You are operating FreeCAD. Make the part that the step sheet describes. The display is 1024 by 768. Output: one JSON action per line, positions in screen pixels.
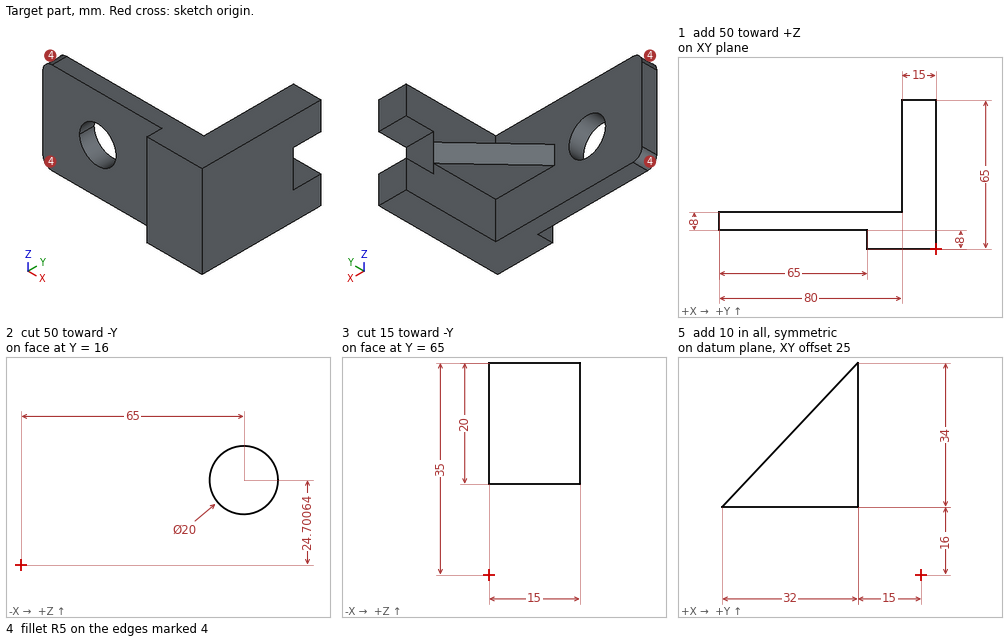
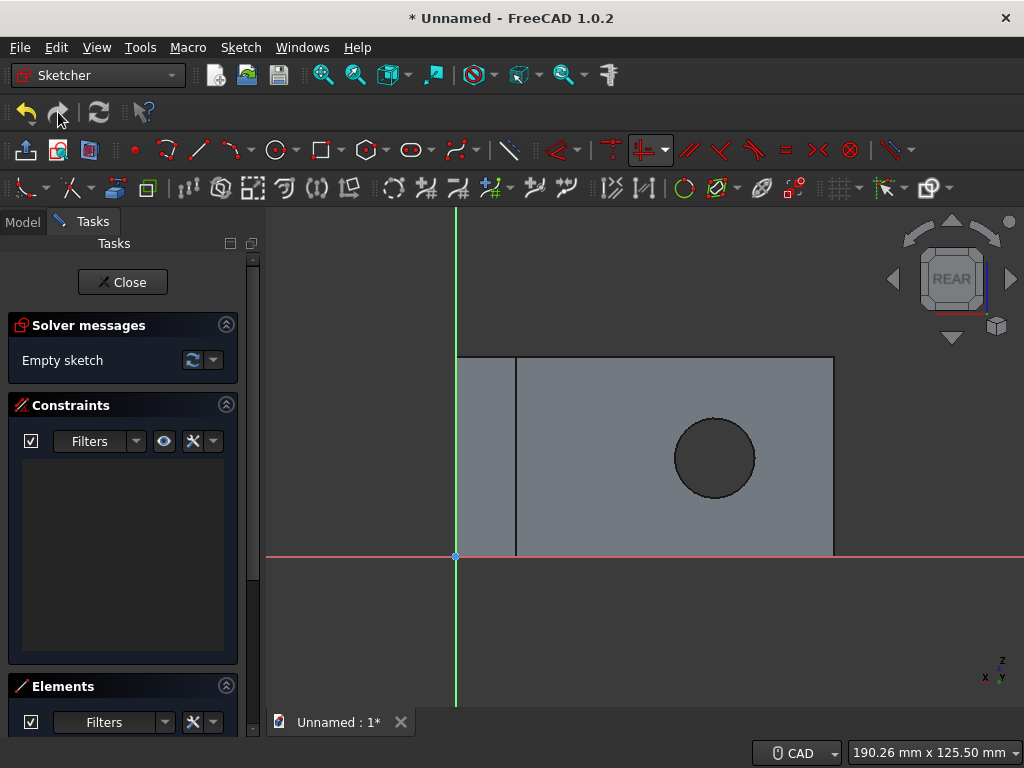
{"action": "scroll", "coordinate": [411, 511], "scroll_direction": "up", "scroll_amount": 4}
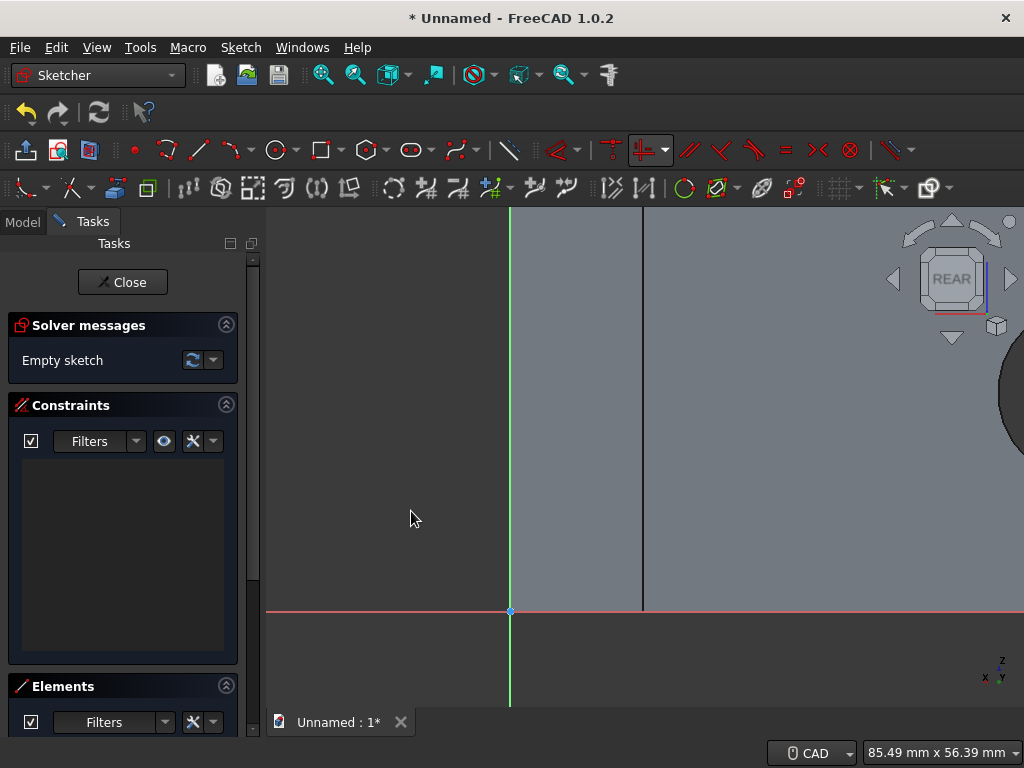
{"action": "left_click", "coordinate": [322, 150]}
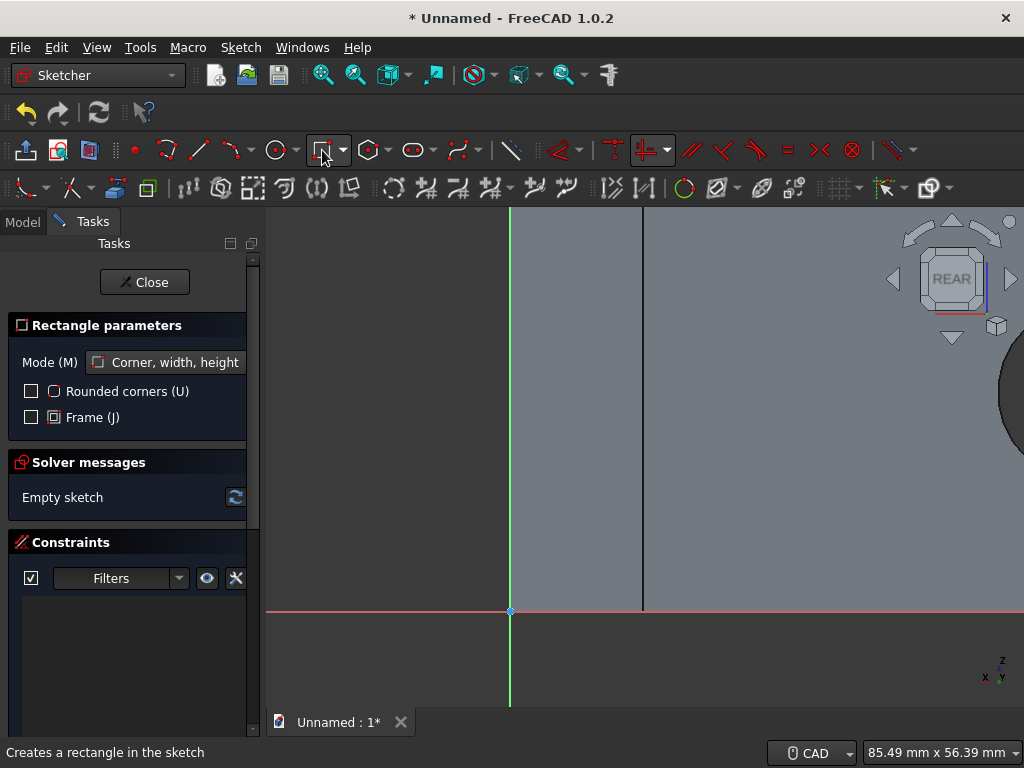
{"action": "left_click", "coordinate": [510, 301]}
{"action": "left_click", "coordinate": [643, 479]}
{"action": "key", "text": "Escape"}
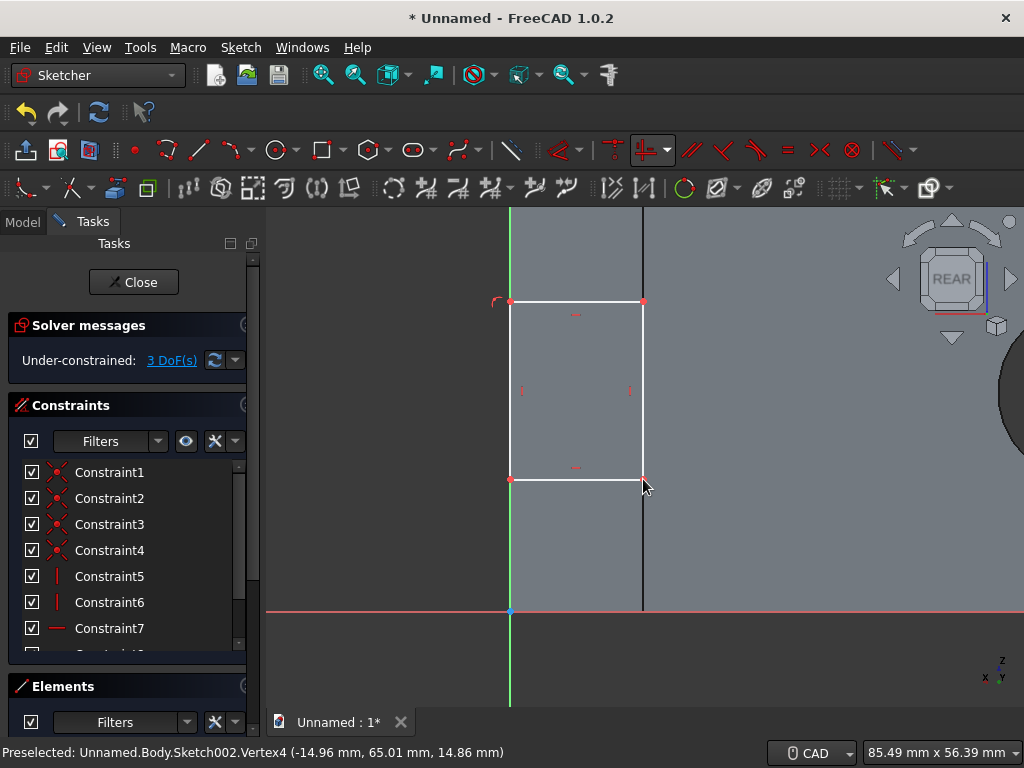
{"action": "left_click", "coordinate": [558, 150]}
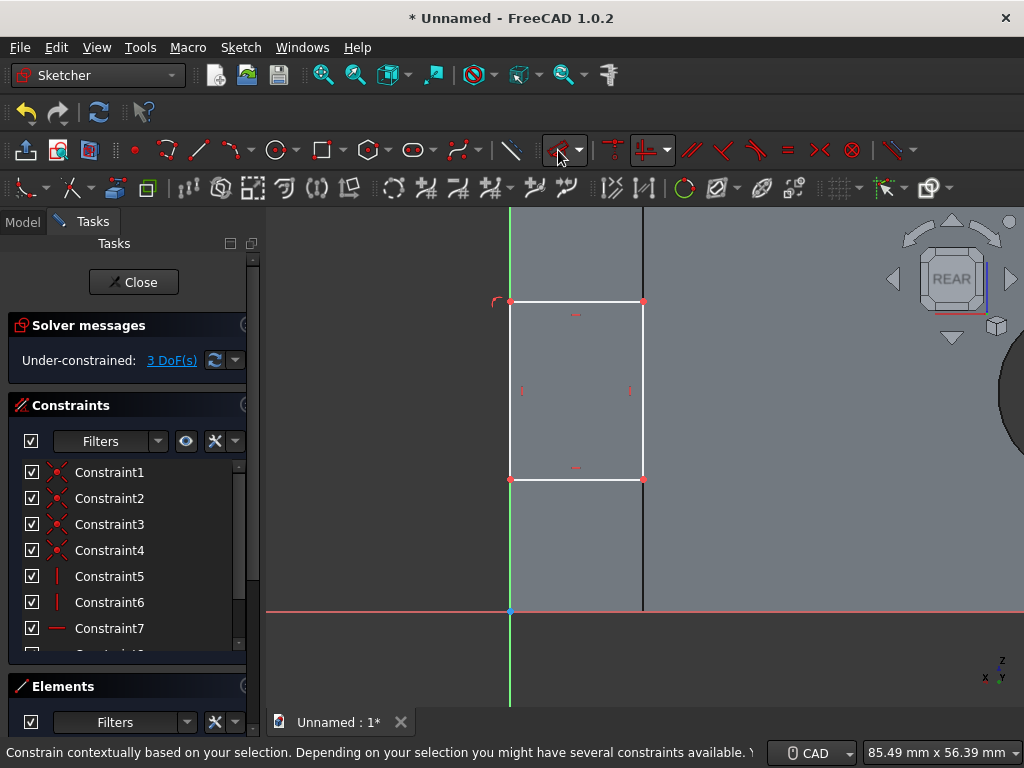
{"action": "left_click", "coordinate": [510, 355]}
{"action": "left_click", "coordinate": [476, 391]}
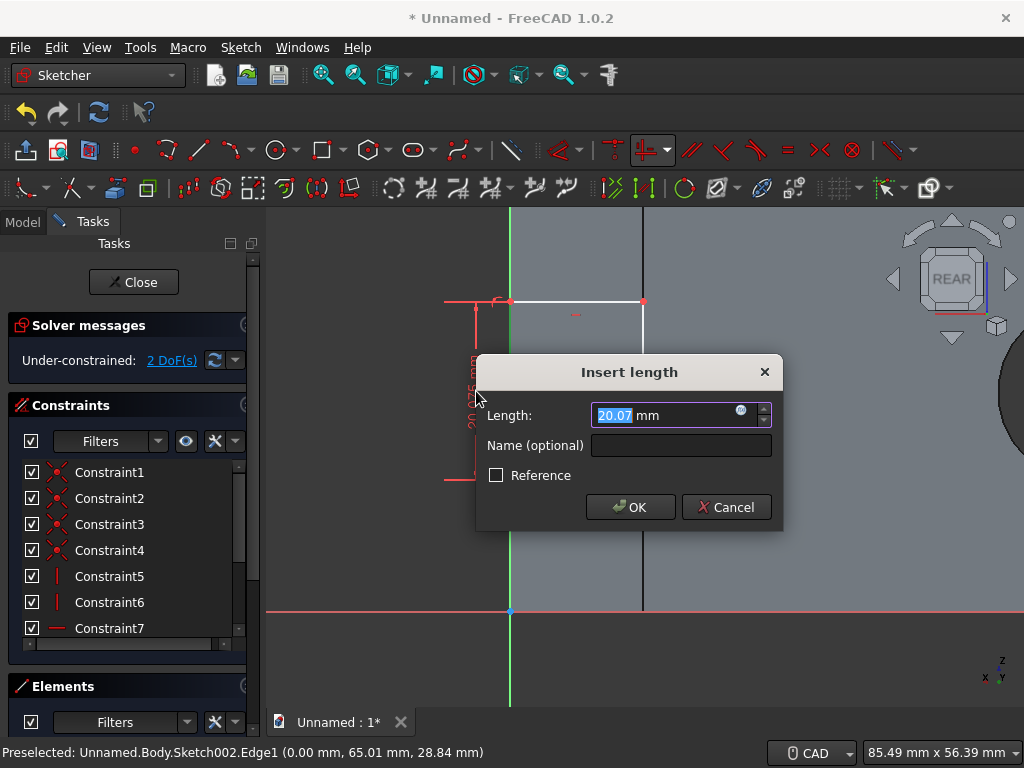
{"action": "type", "text": "20"}
{"action": "key", "text": "Return"}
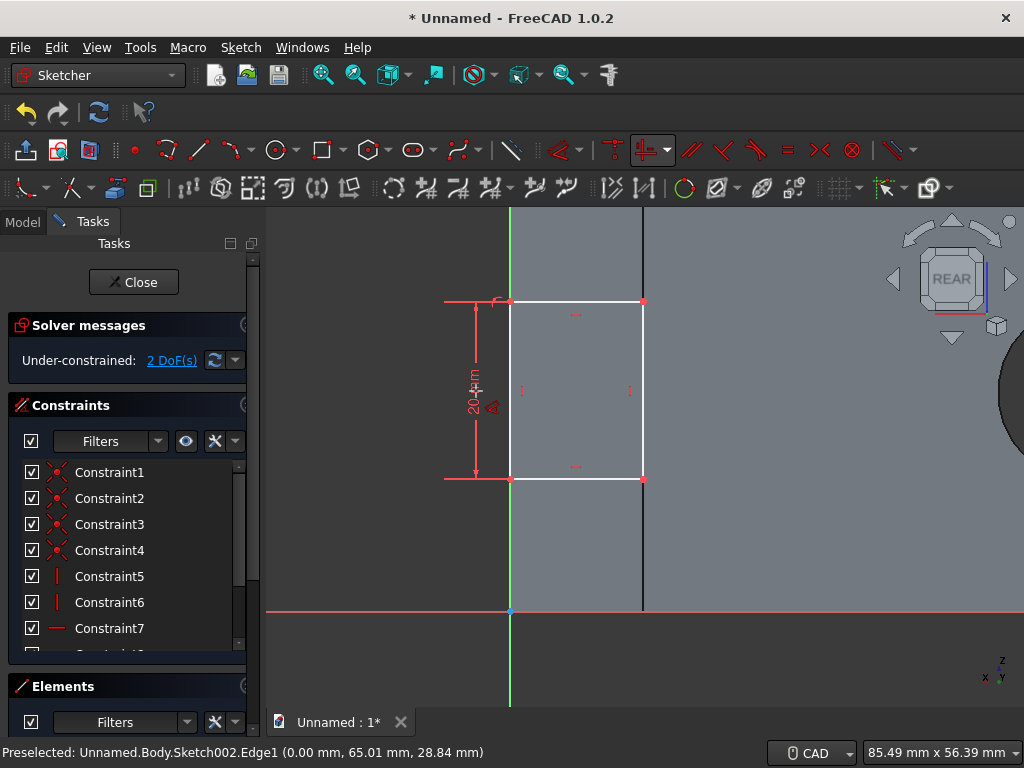
{"action": "left_click", "coordinate": [550, 479]}
{"action": "left_click", "coordinate": [577, 513]}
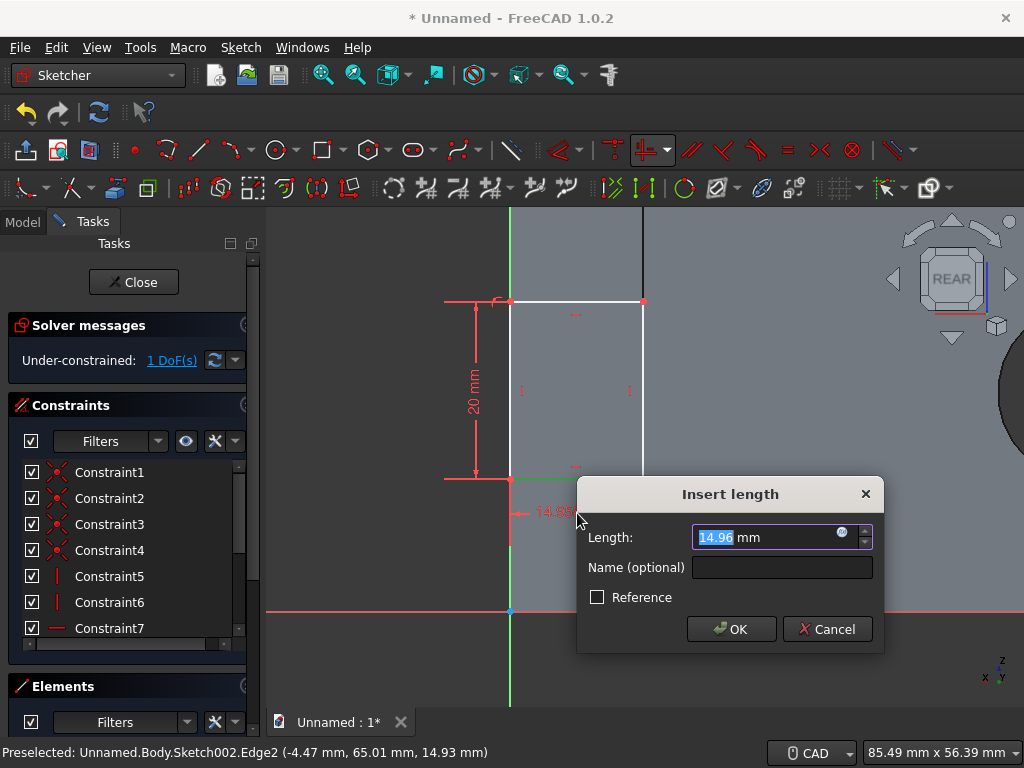
{"action": "type", "text": "15"}
{"action": "key", "text": "Return"}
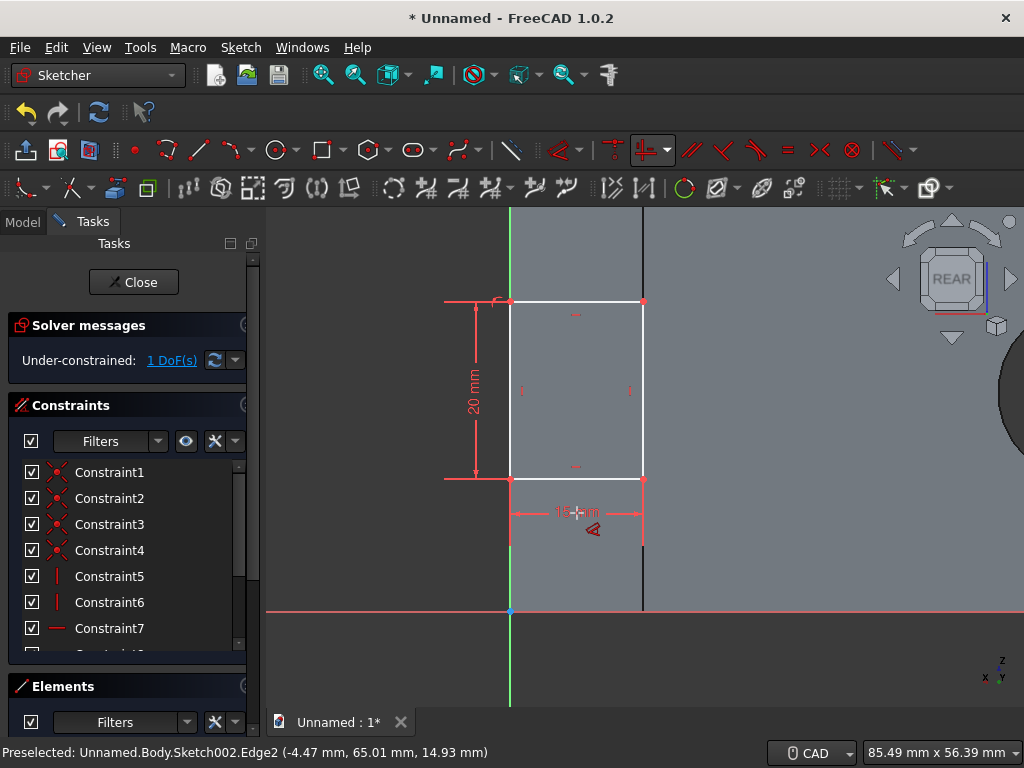
{"action": "left_click", "coordinate": [510, 302]}
{"action": "left_click", "coordinate": [476, 457]}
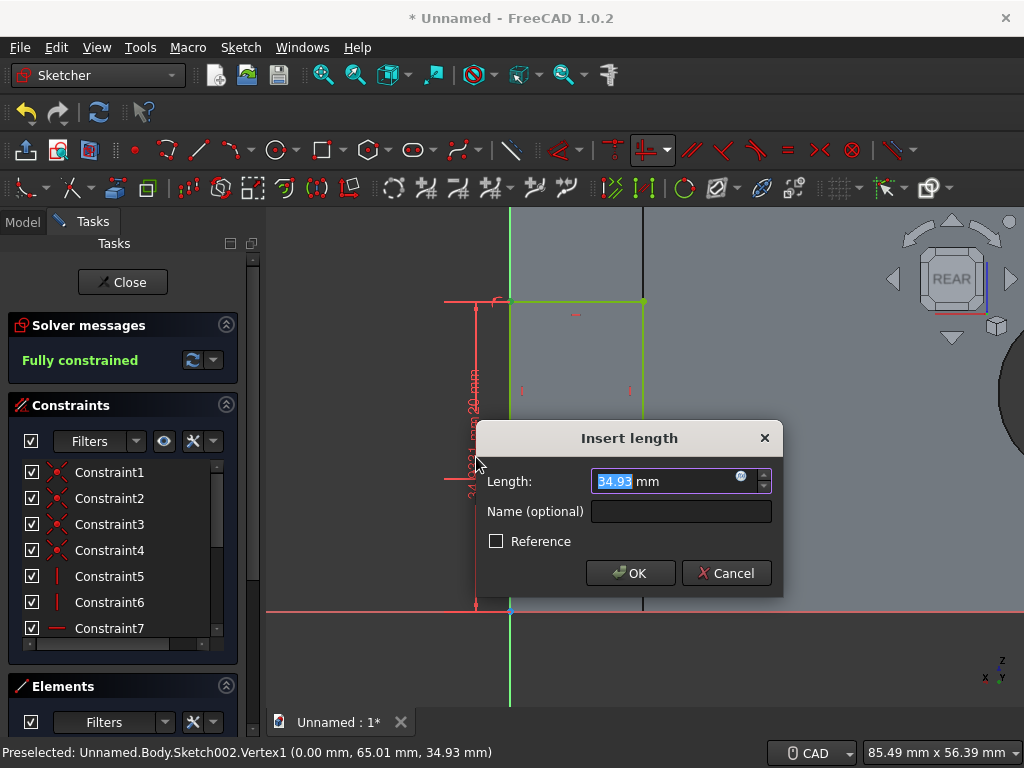
{"action": "type", "text": "35"}
{"action": "key", "text": "Return"}
{"action": "key", "text": "Escape"}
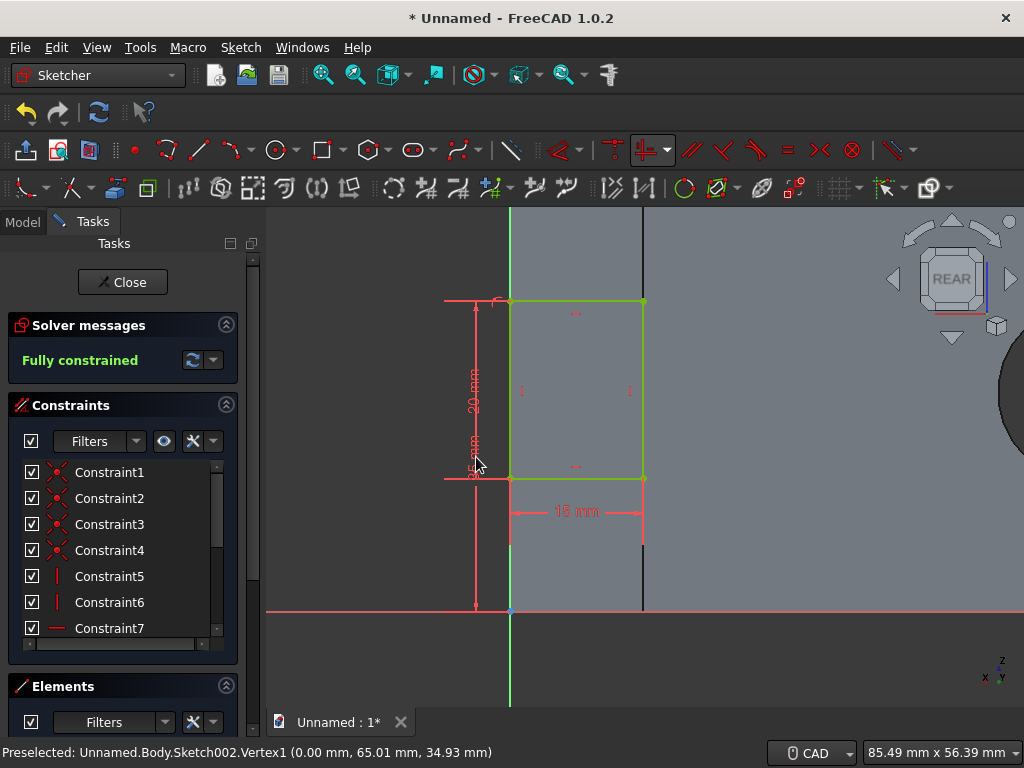
{"action": "left_click", "coordinate": [123, 282]}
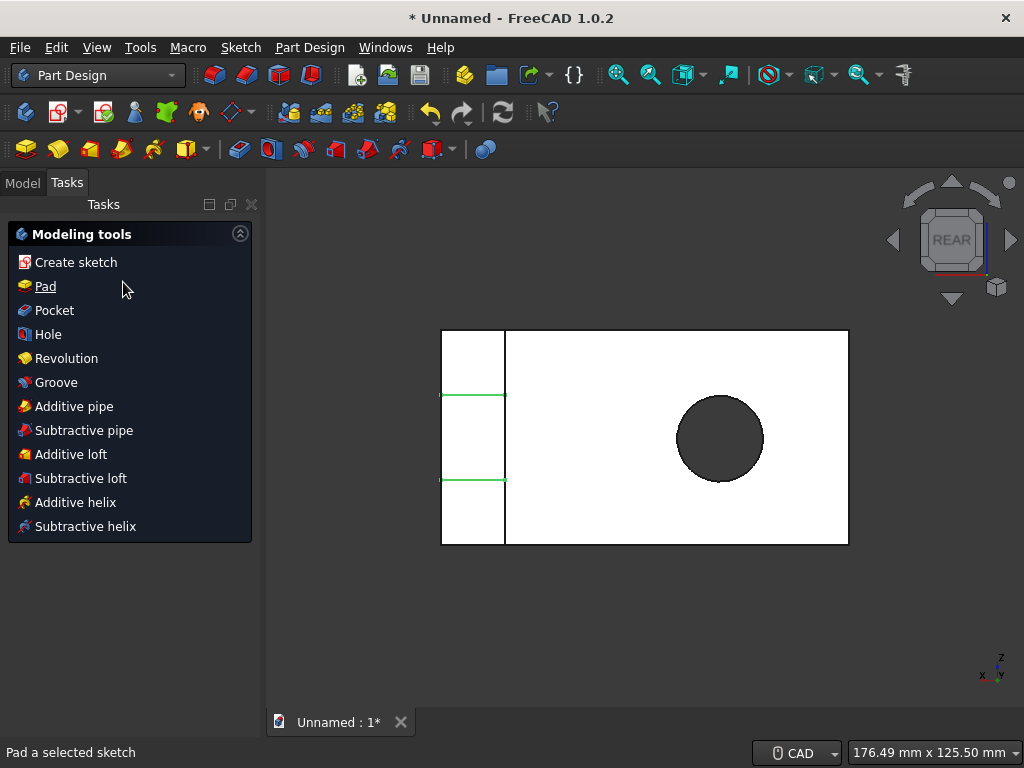
{"action": "left_click", "coordinate": [240, 150]}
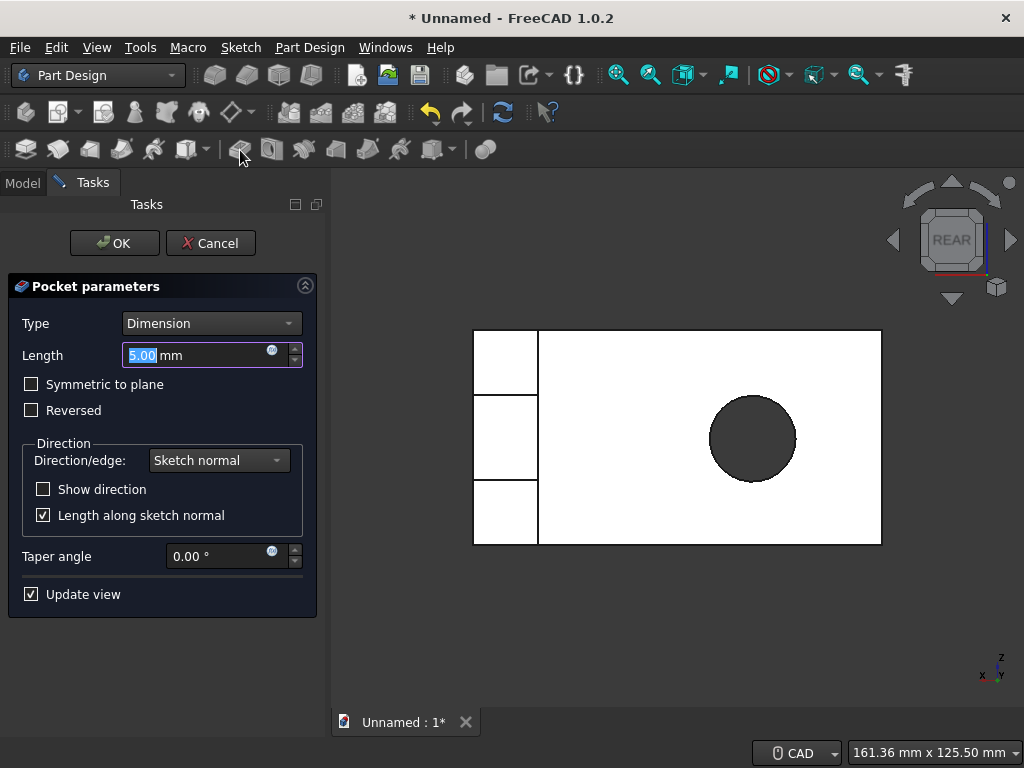
{"action": "type", "text": "15"}
{"action": "key", "text": "Tab"}